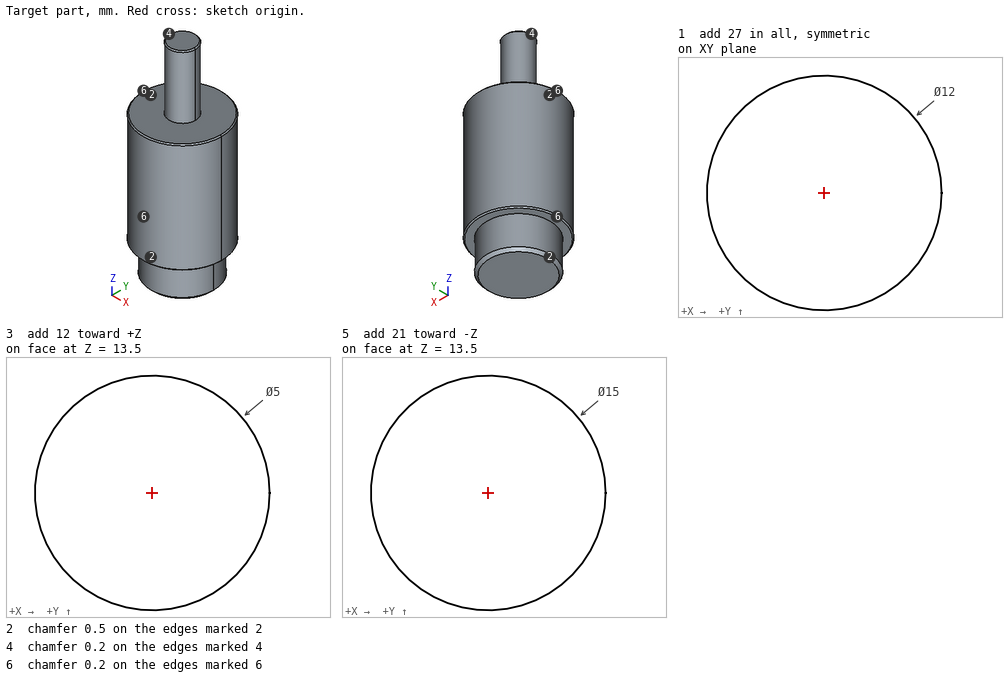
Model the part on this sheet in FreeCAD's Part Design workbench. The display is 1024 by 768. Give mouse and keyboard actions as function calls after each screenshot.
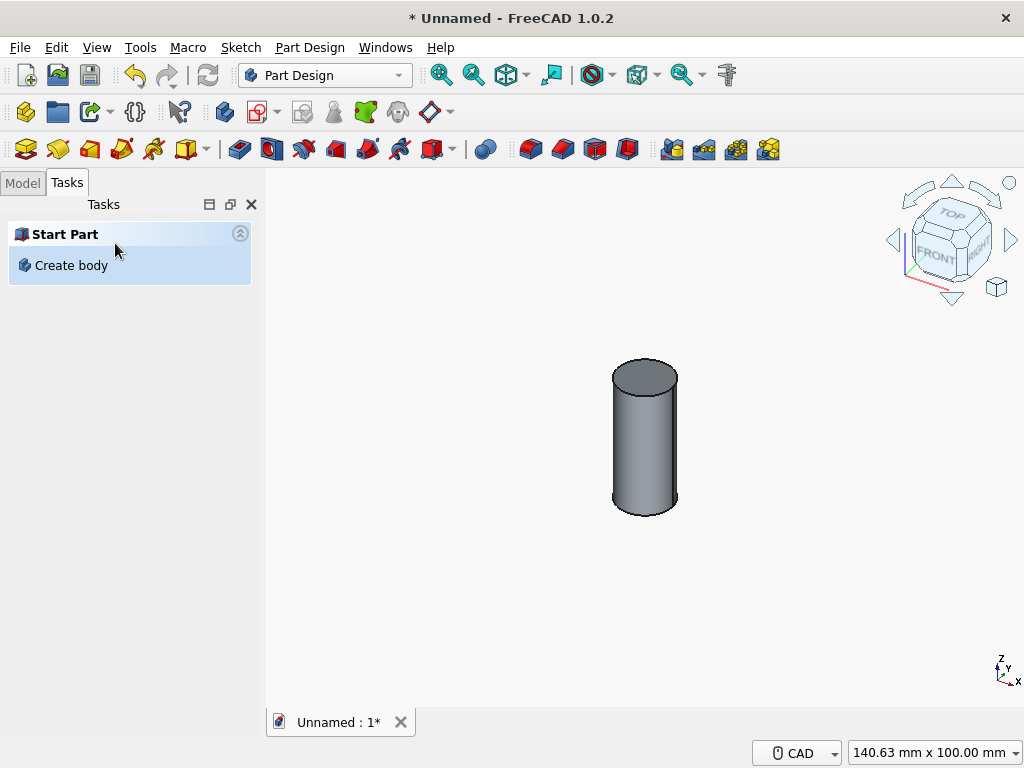
click(442, 76)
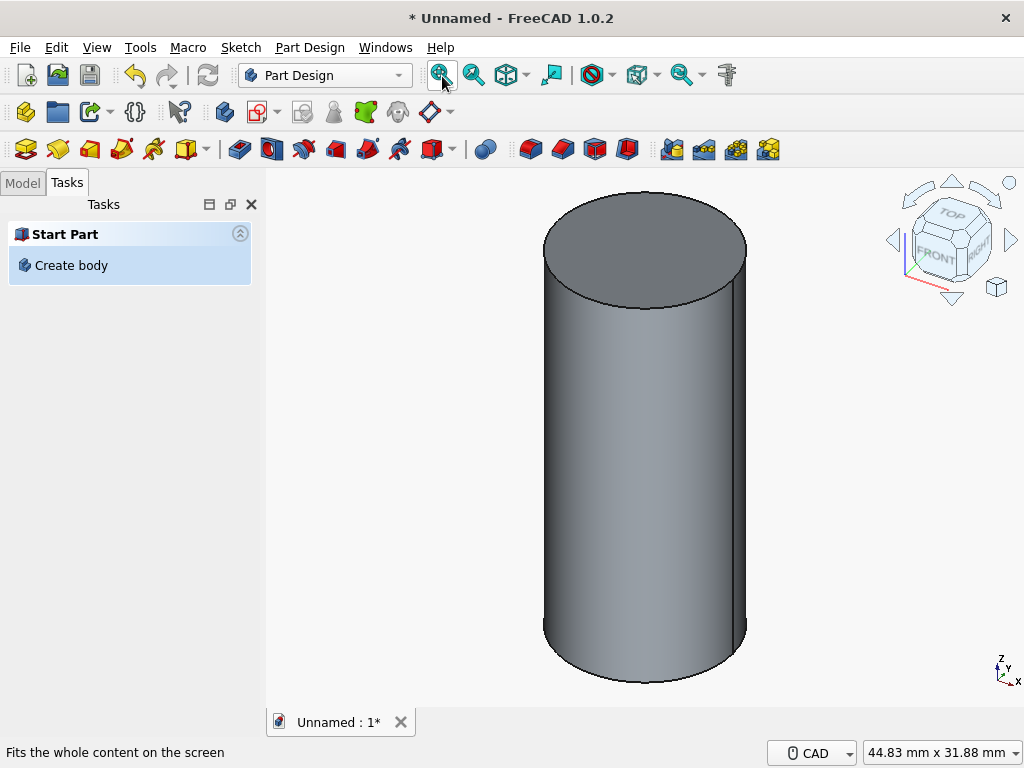
click(741, 643)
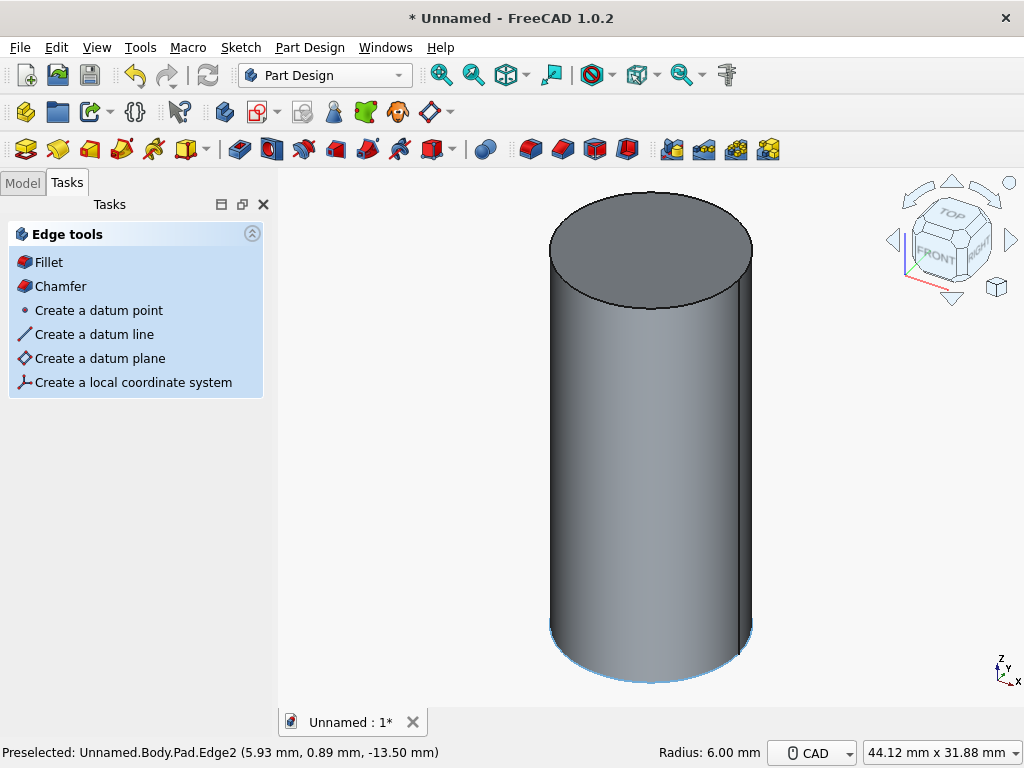
click(550, 256, ctrl)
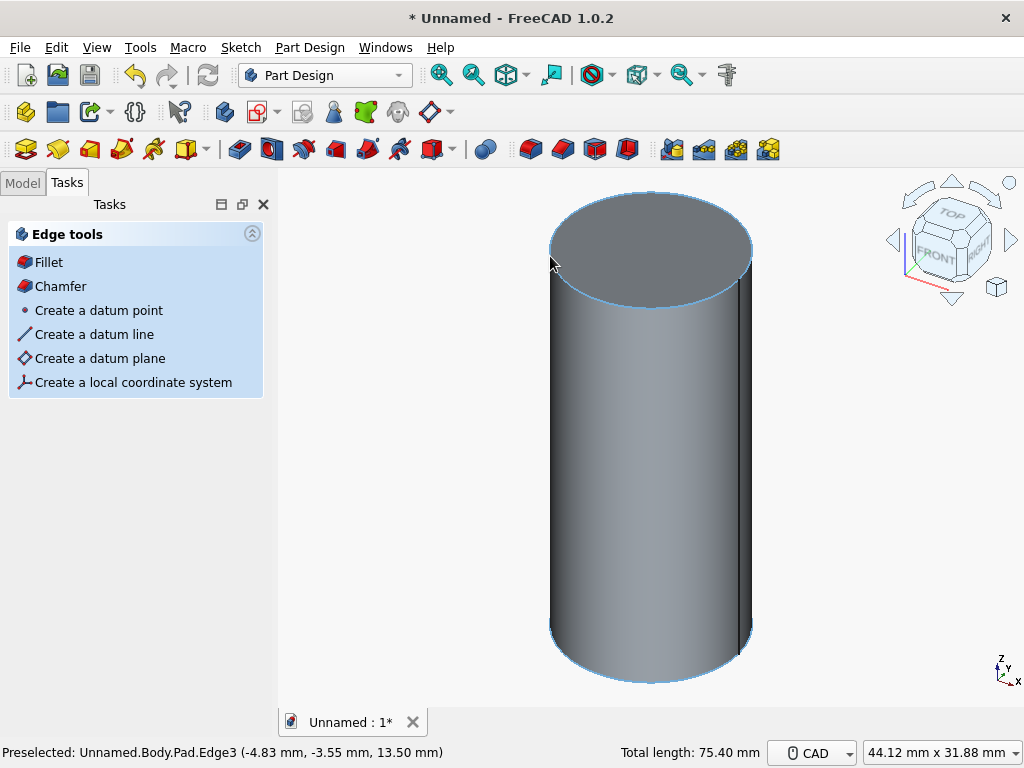
click(564, 150)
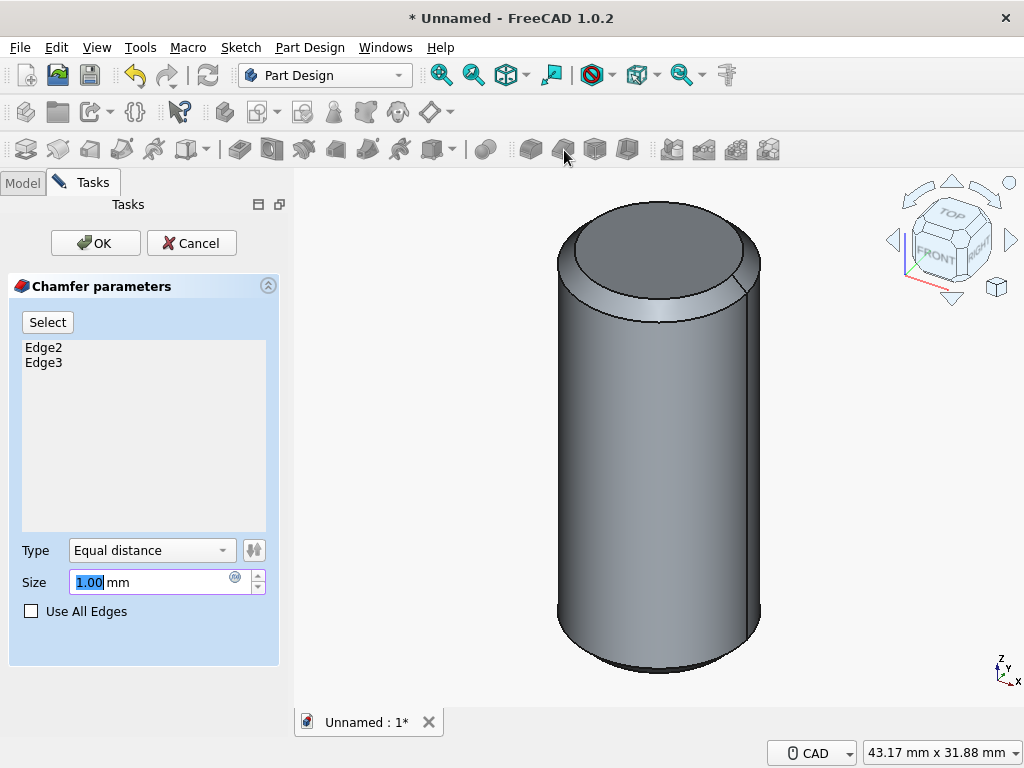
text(0.5)
key(Tab)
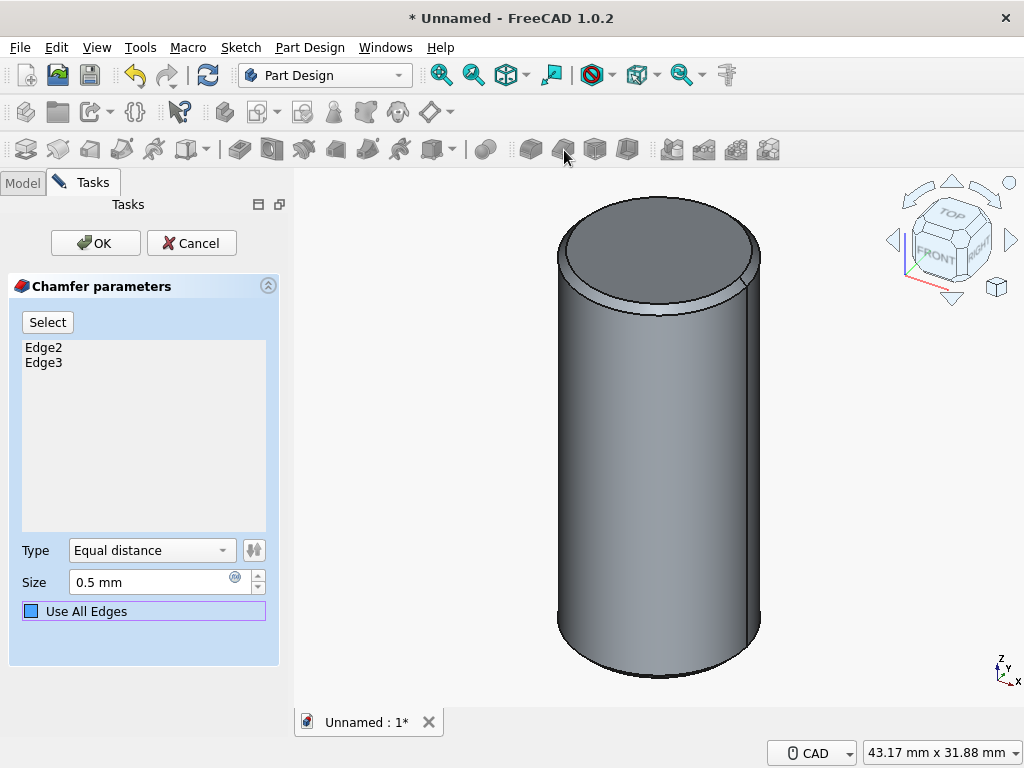
click(96, 243)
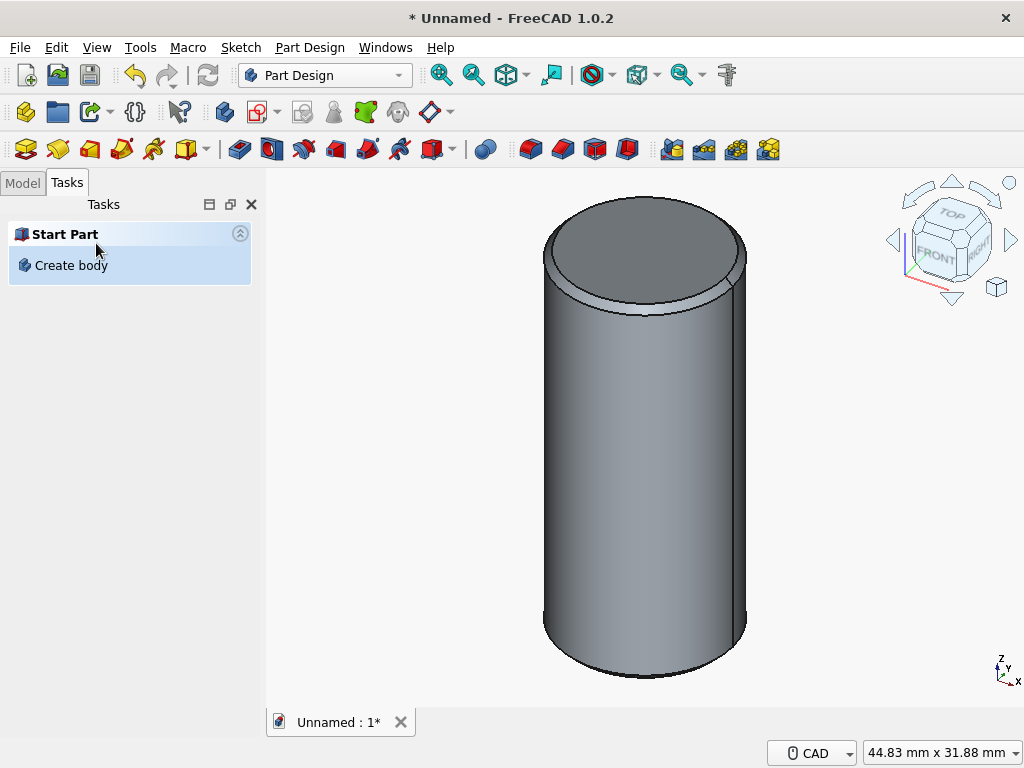
click(645, 250)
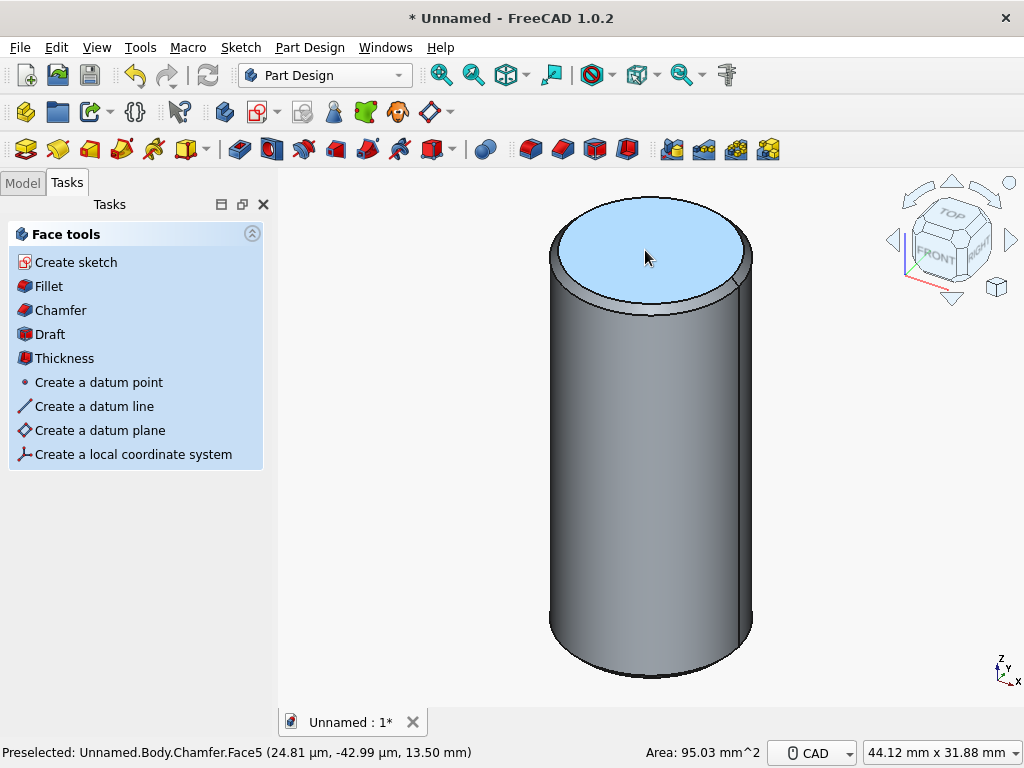
click(258, 112)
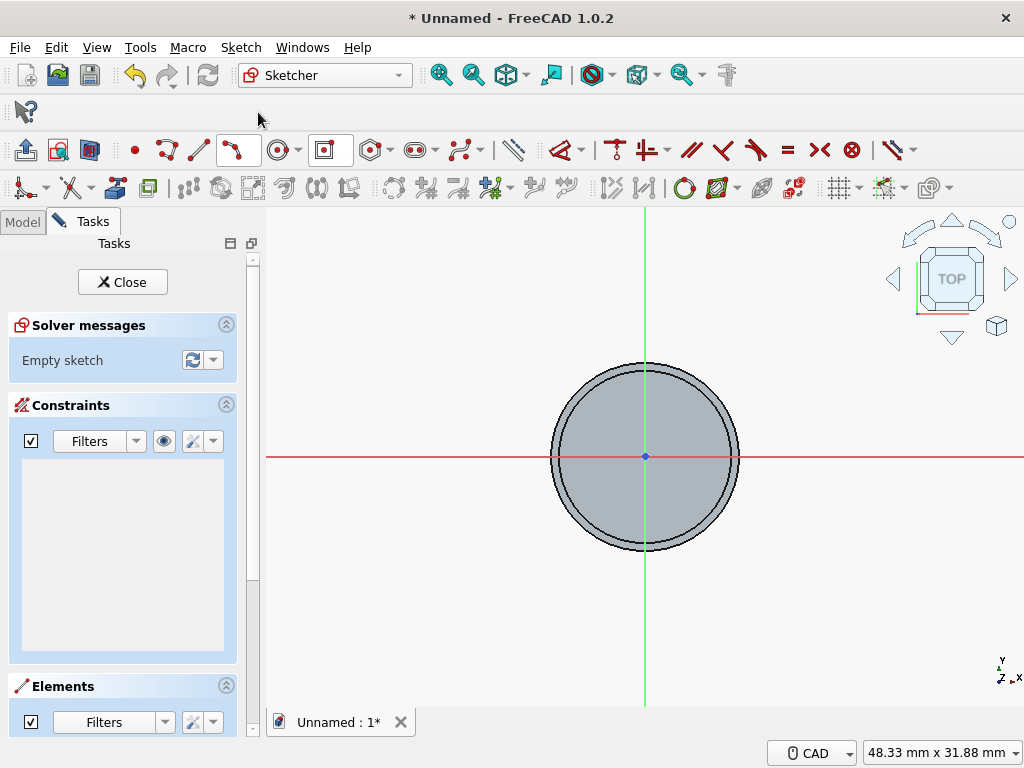
scroll(667, 457, up, 7)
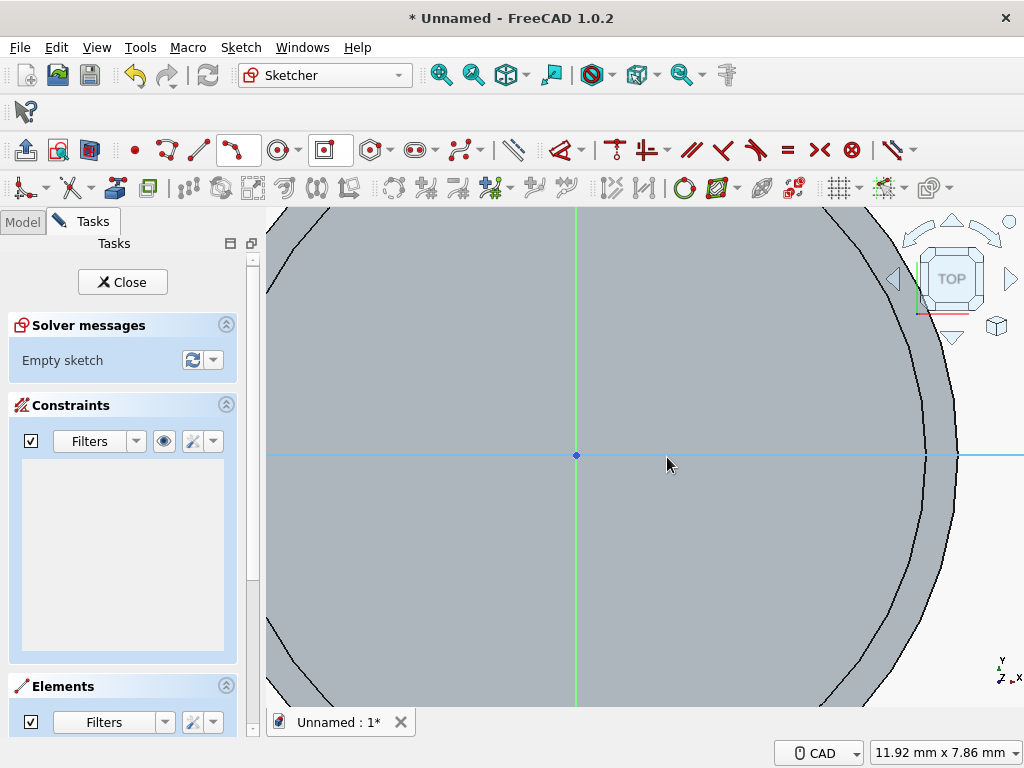
click(278, 150)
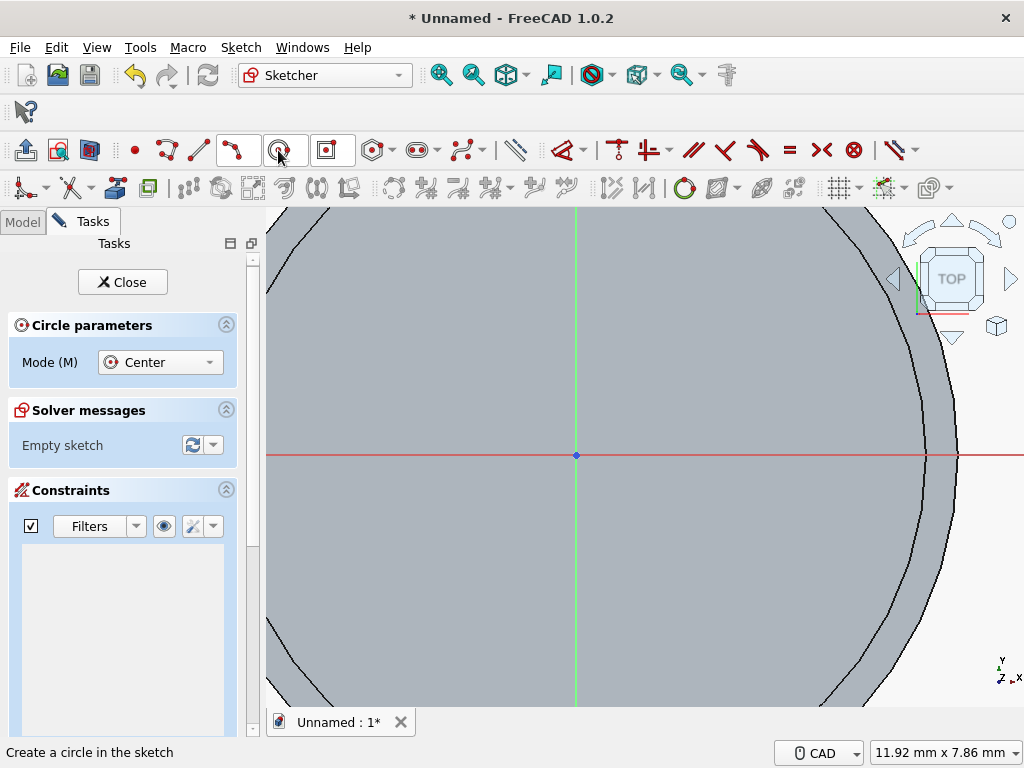
click(576, 455)
move(689, 343)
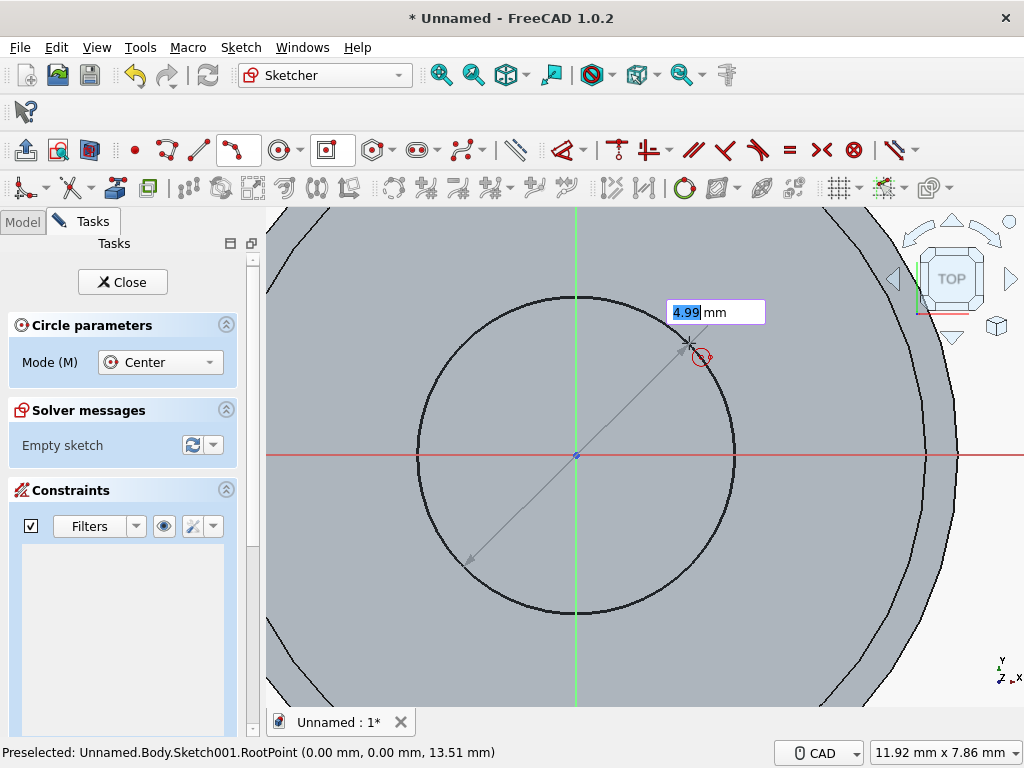
text(5)
key(Return)
key(Escape)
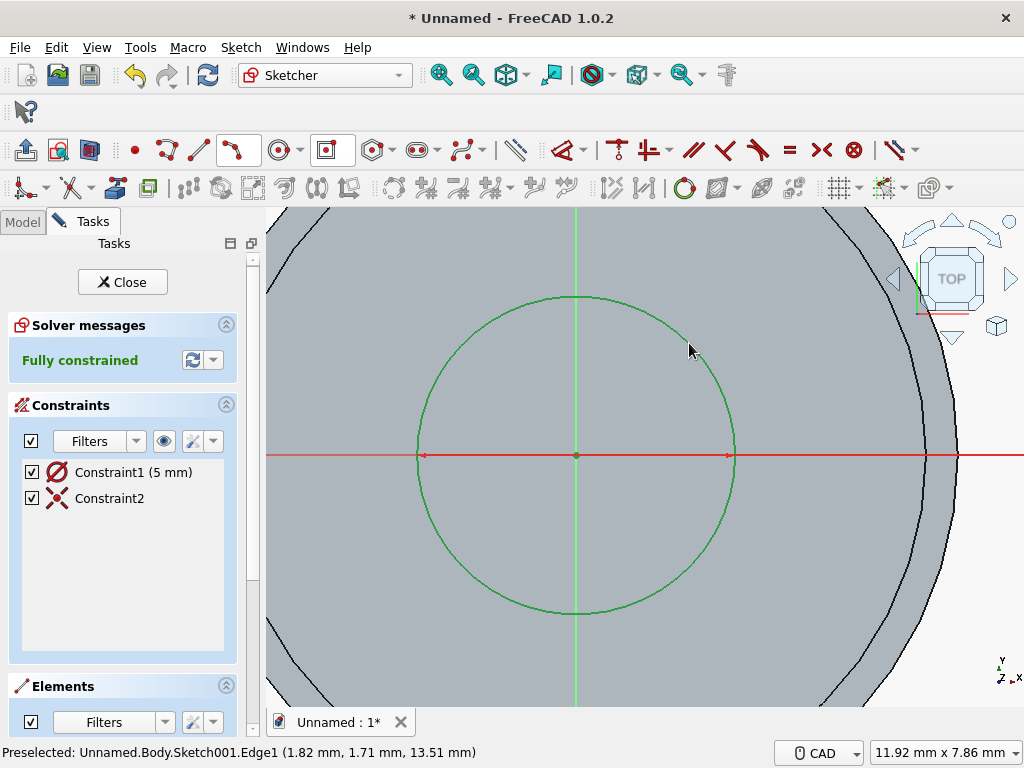
click(123, 282)